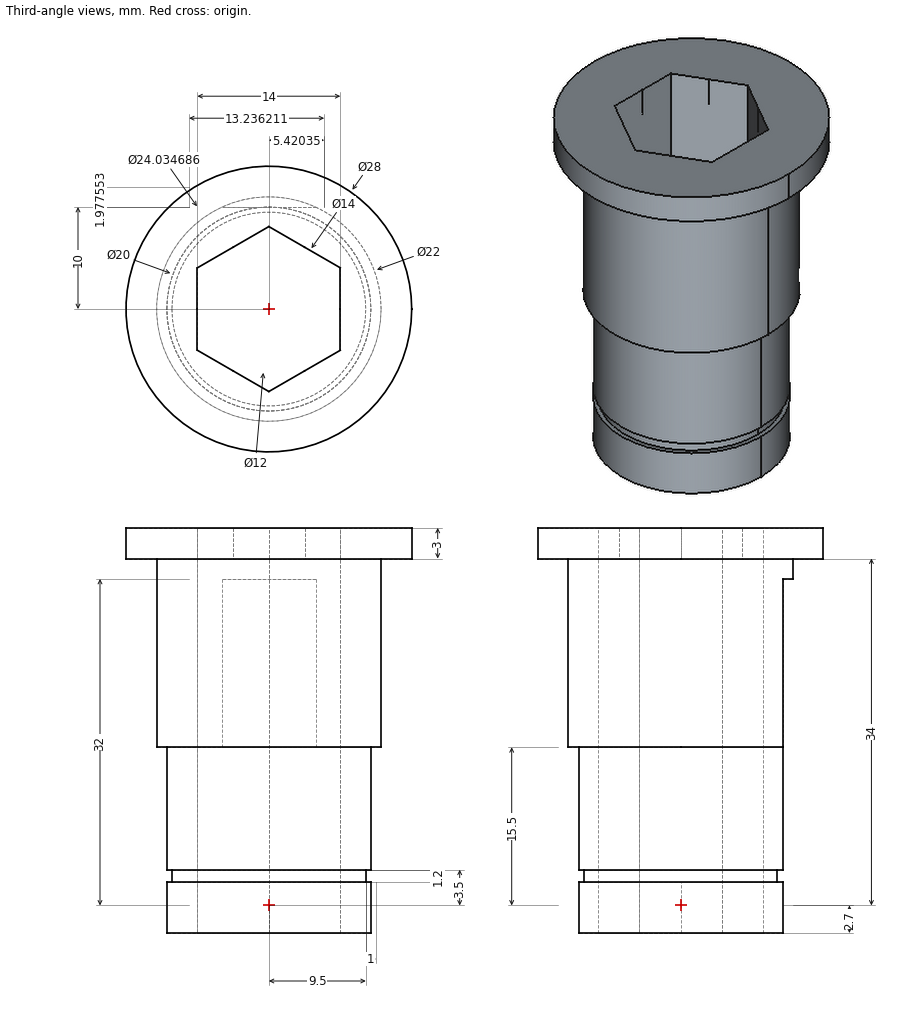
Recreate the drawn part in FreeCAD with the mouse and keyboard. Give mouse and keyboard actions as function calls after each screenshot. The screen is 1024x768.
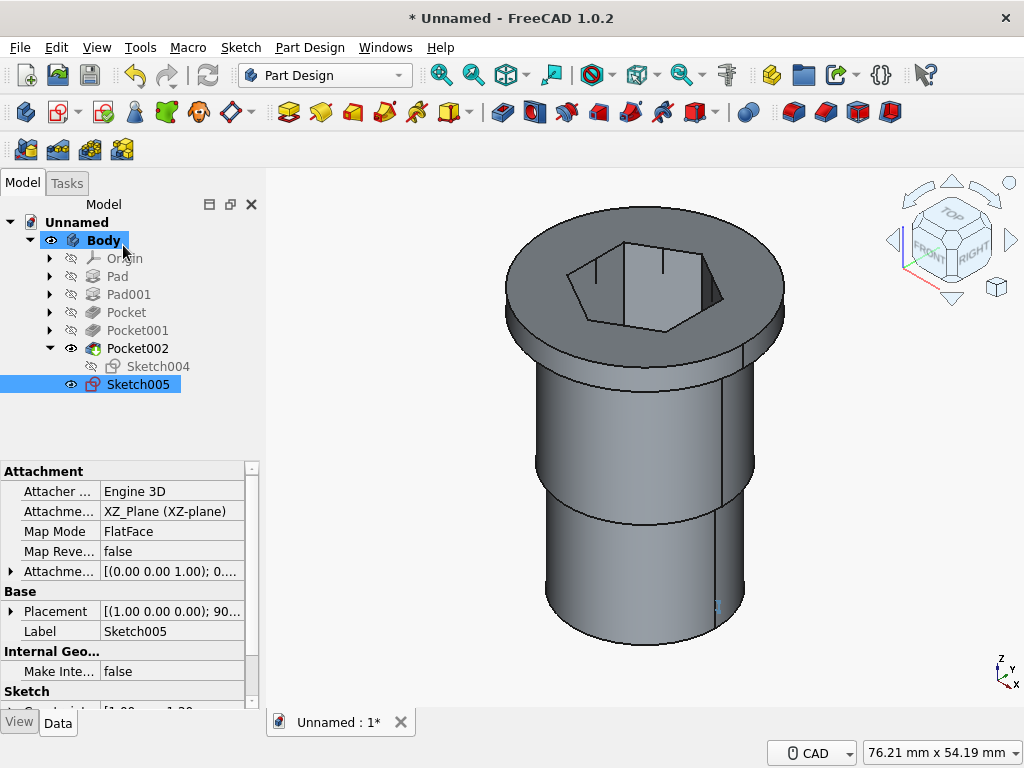
click(568, 112)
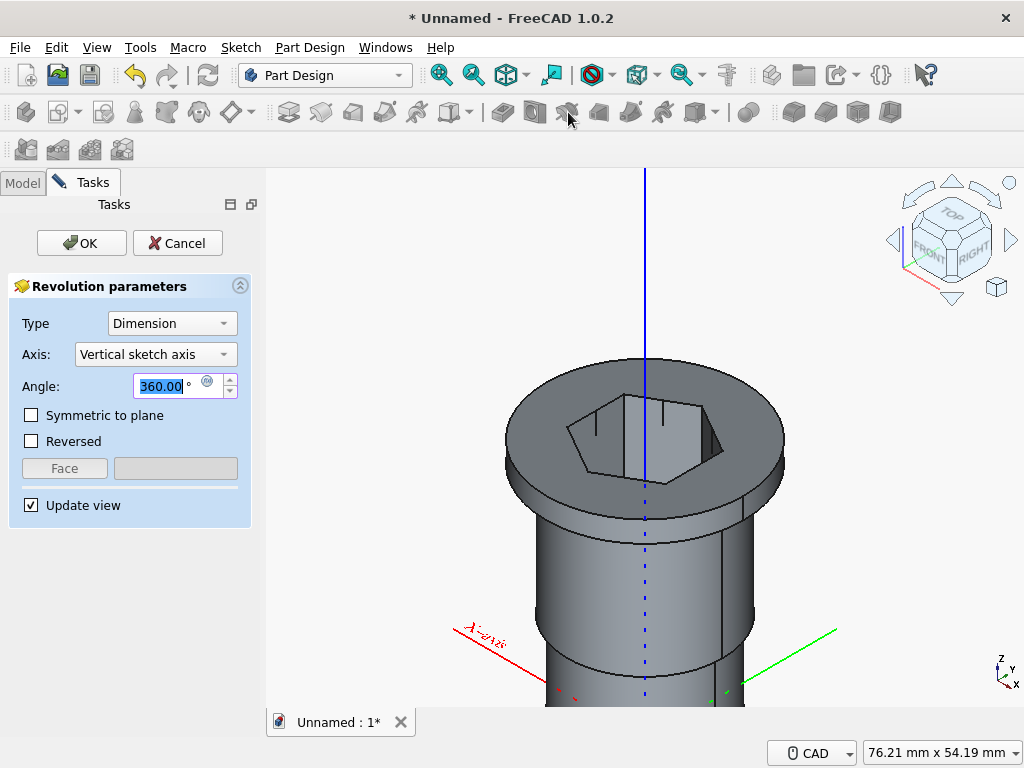
click(82, 243)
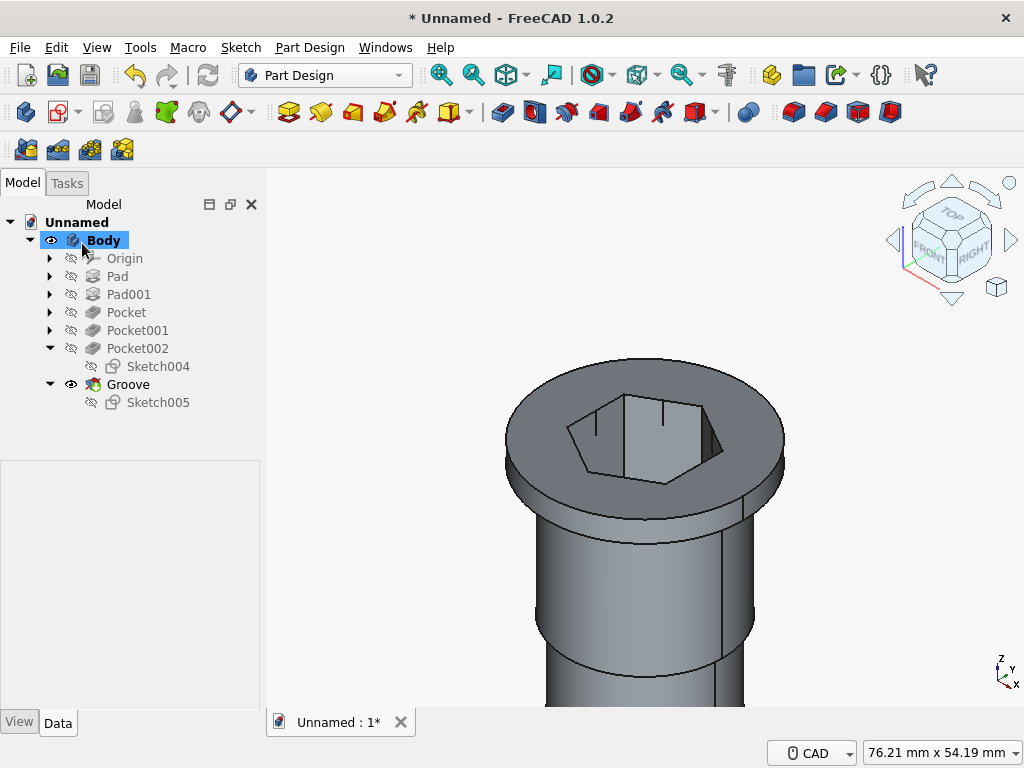
click(442, 76)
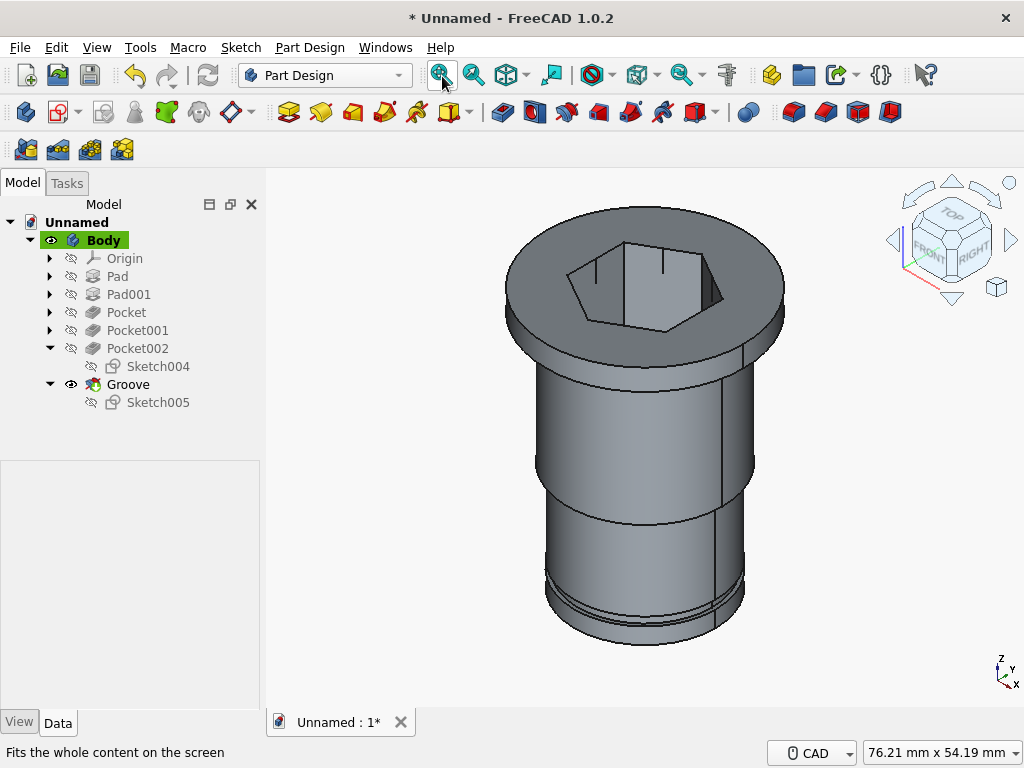
click(50, 258)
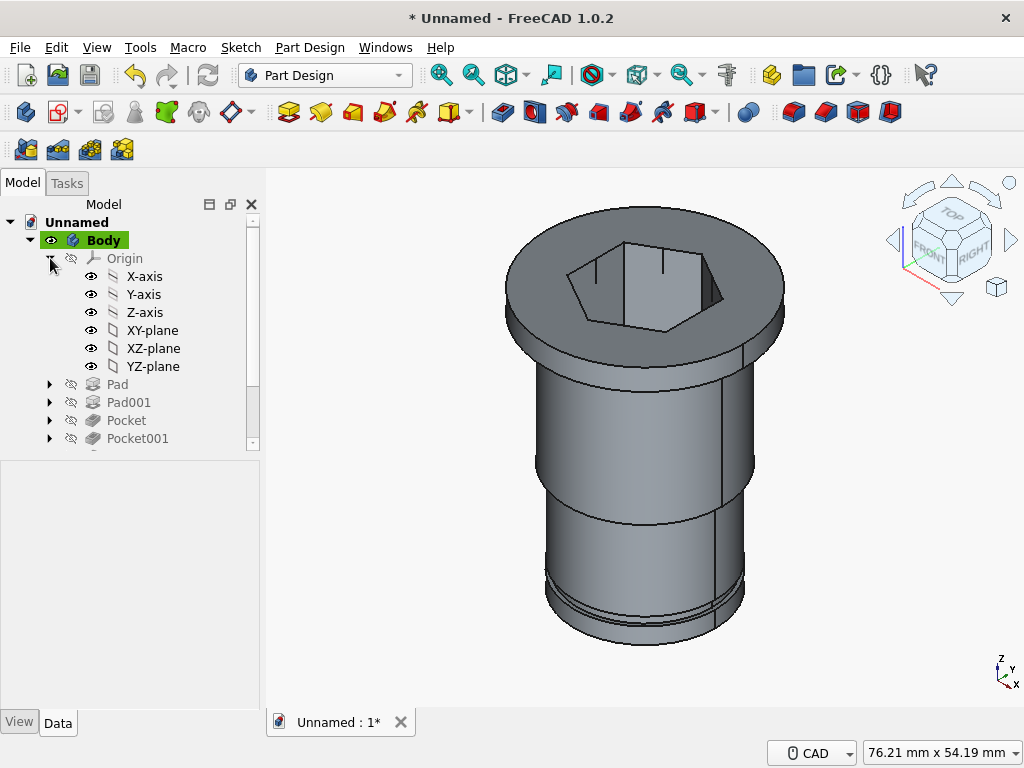
click(136, 330)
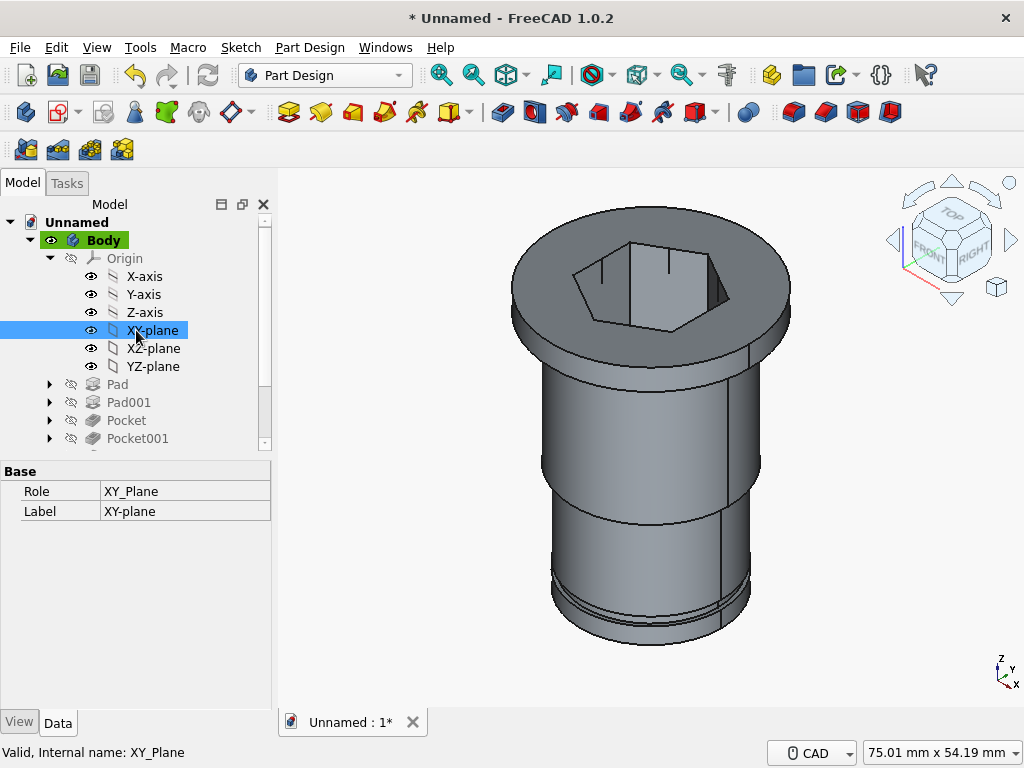
click(232, 112)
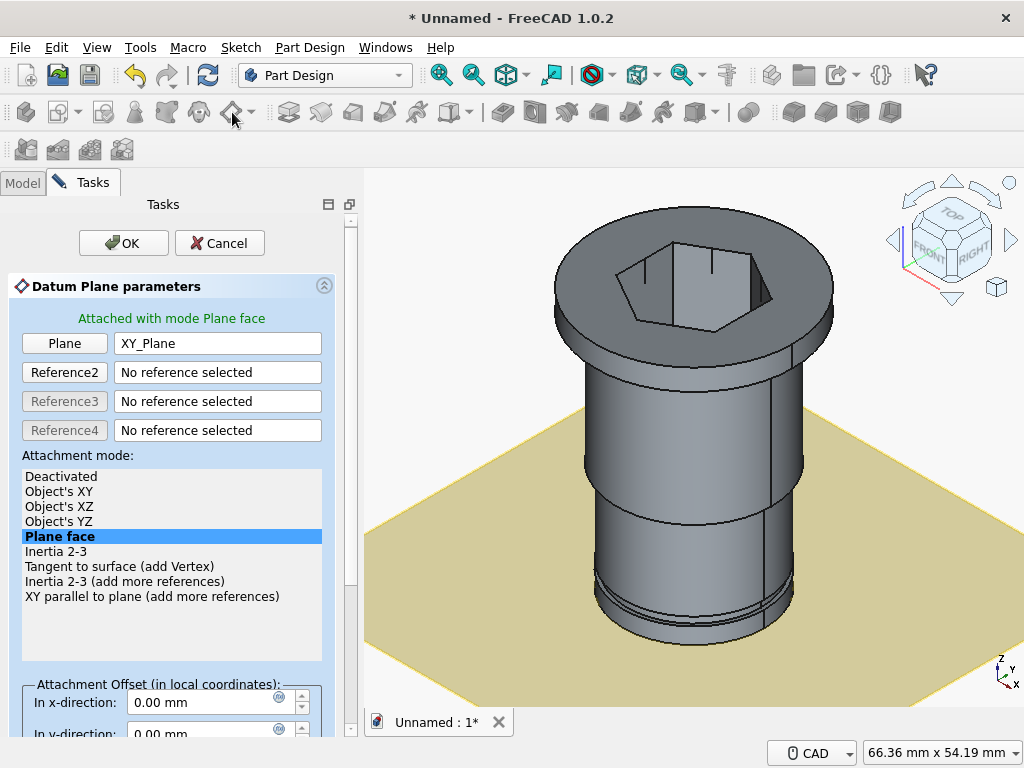
scroll(351, 475, down, 2)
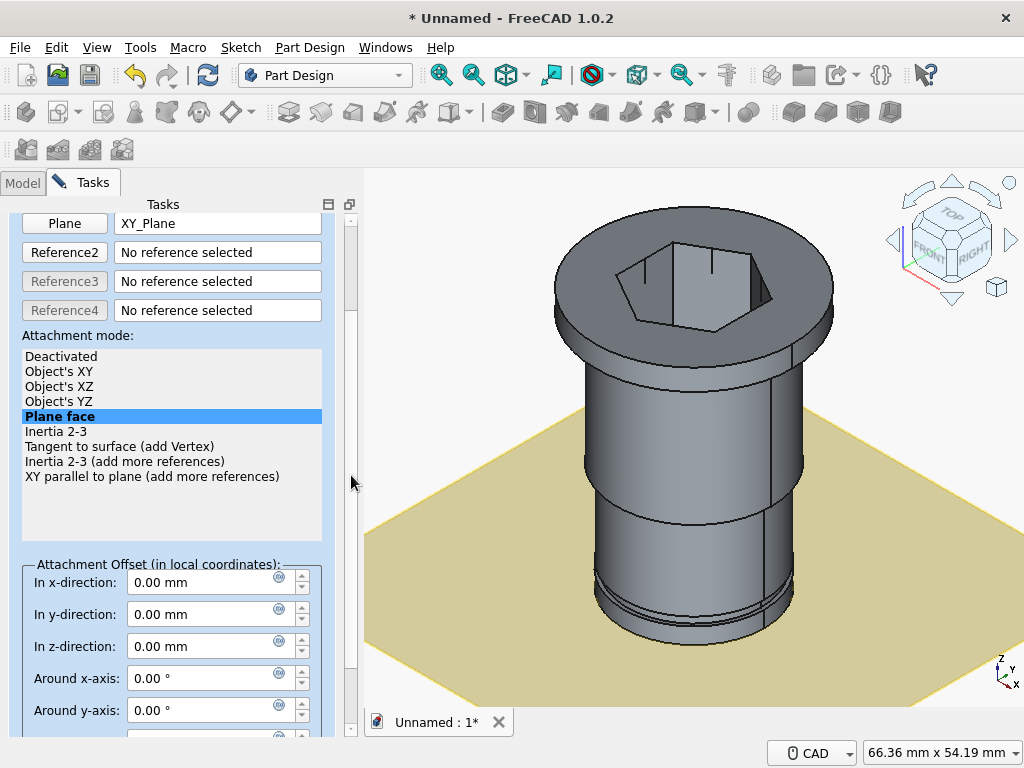
triple_click(210, 646)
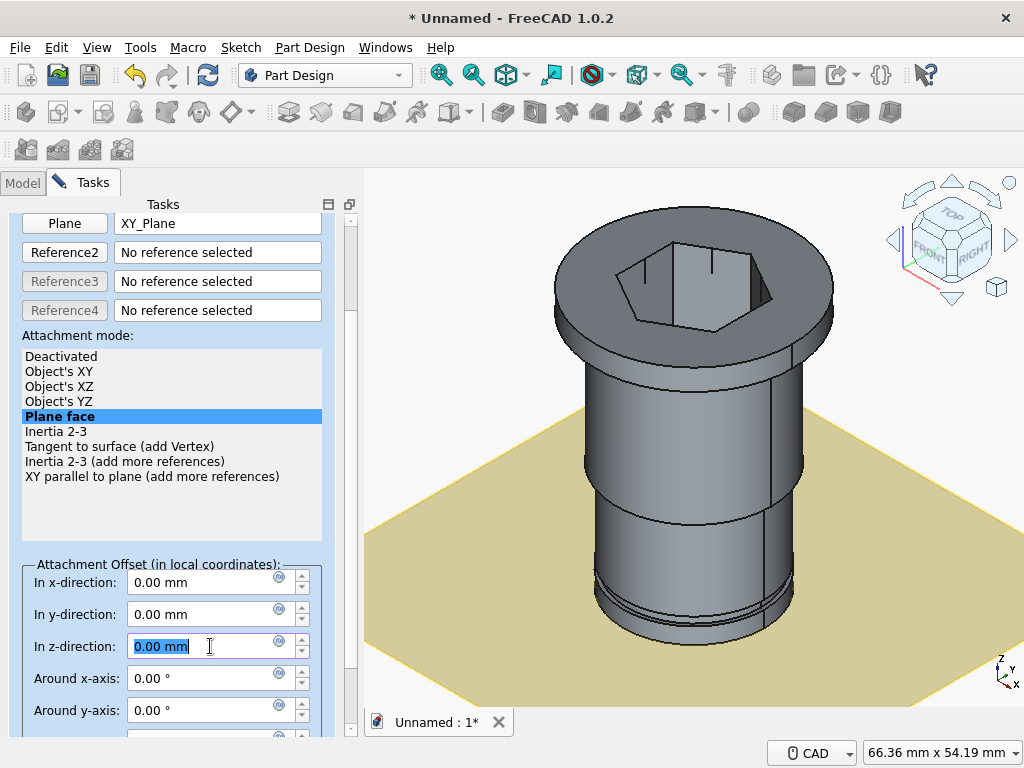
text(-2.7)
key(Tab)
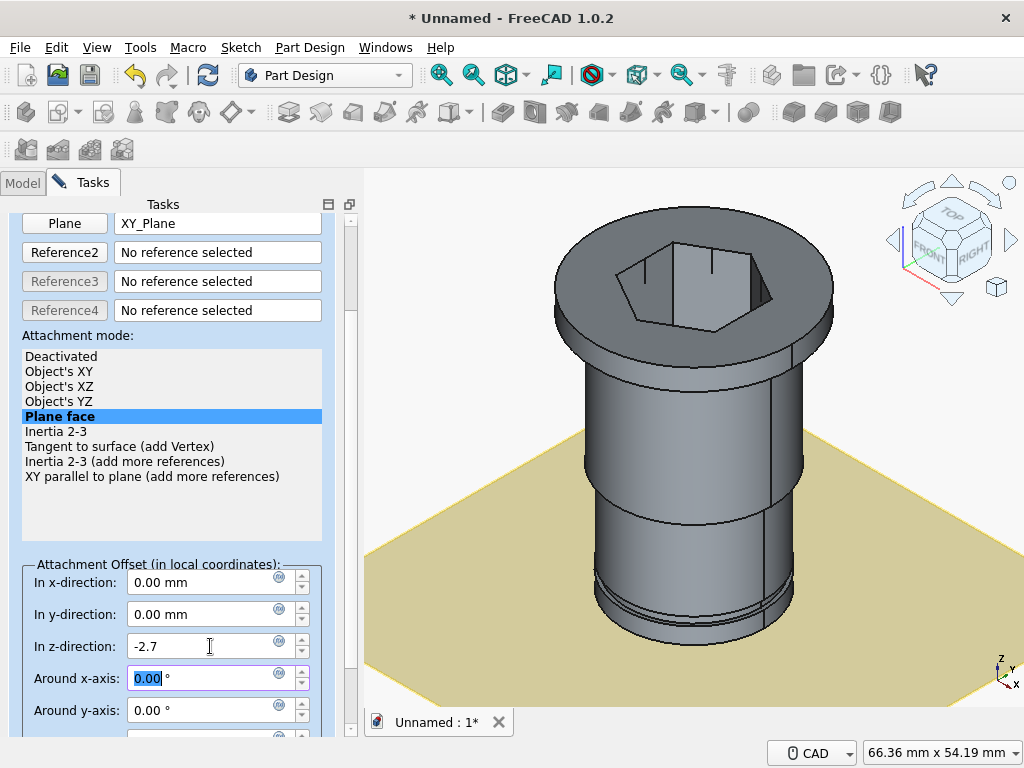
scroll(351, 475, up, 3)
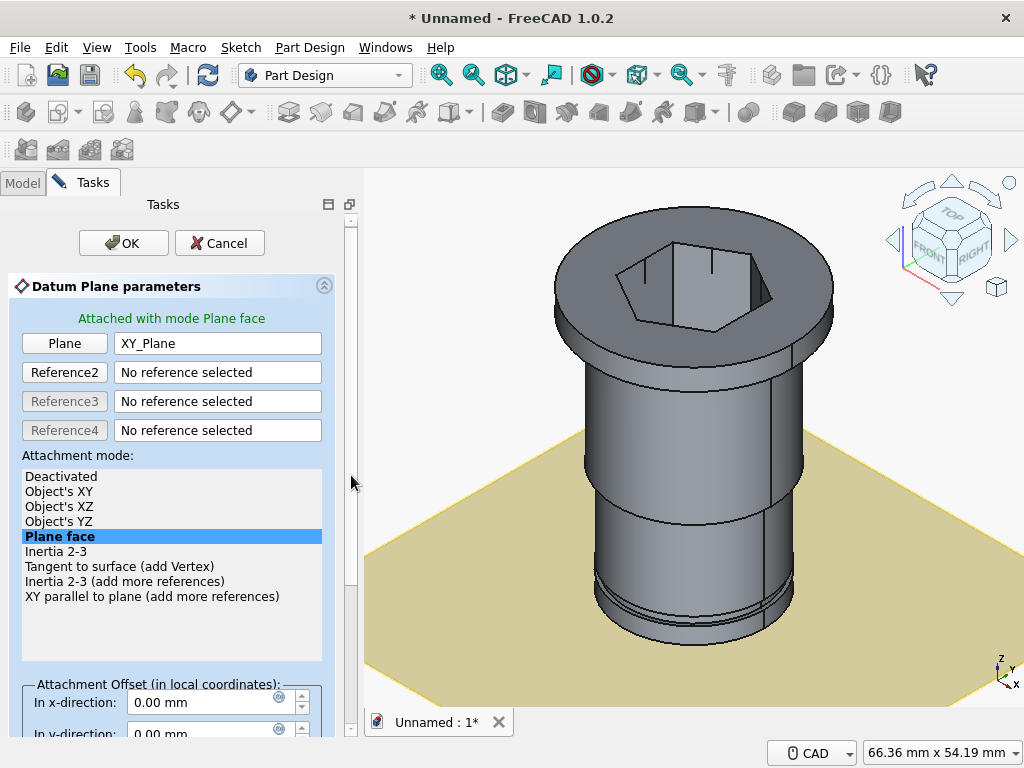
click(124, 243)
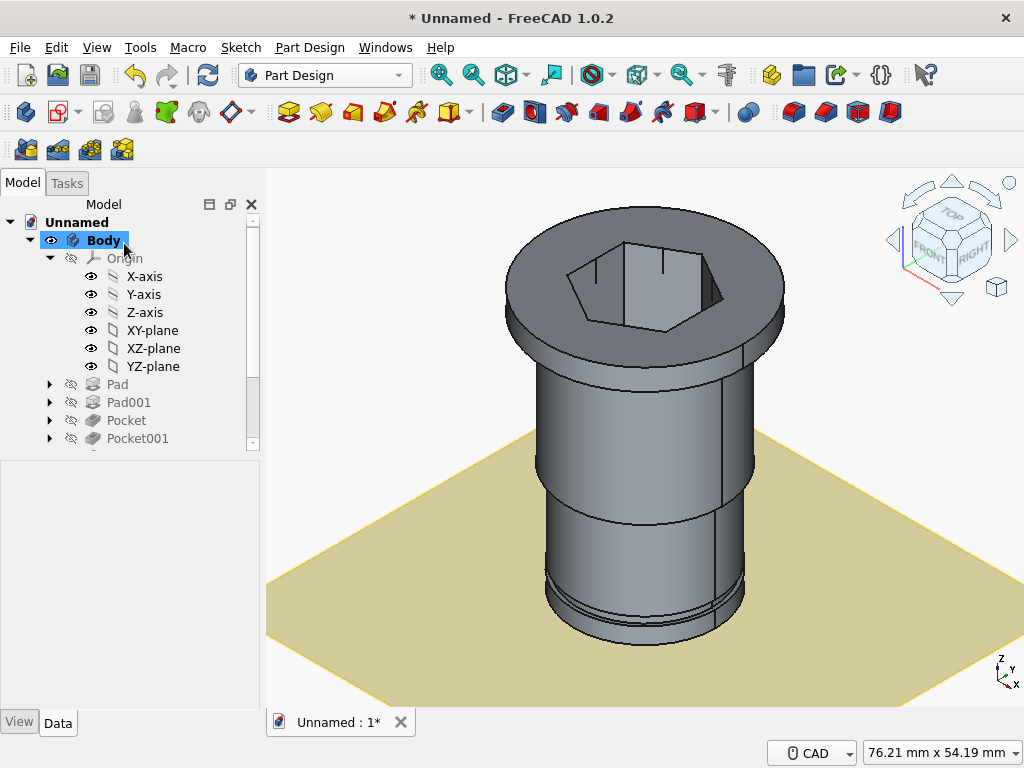
scroll(100, 326, down, 3)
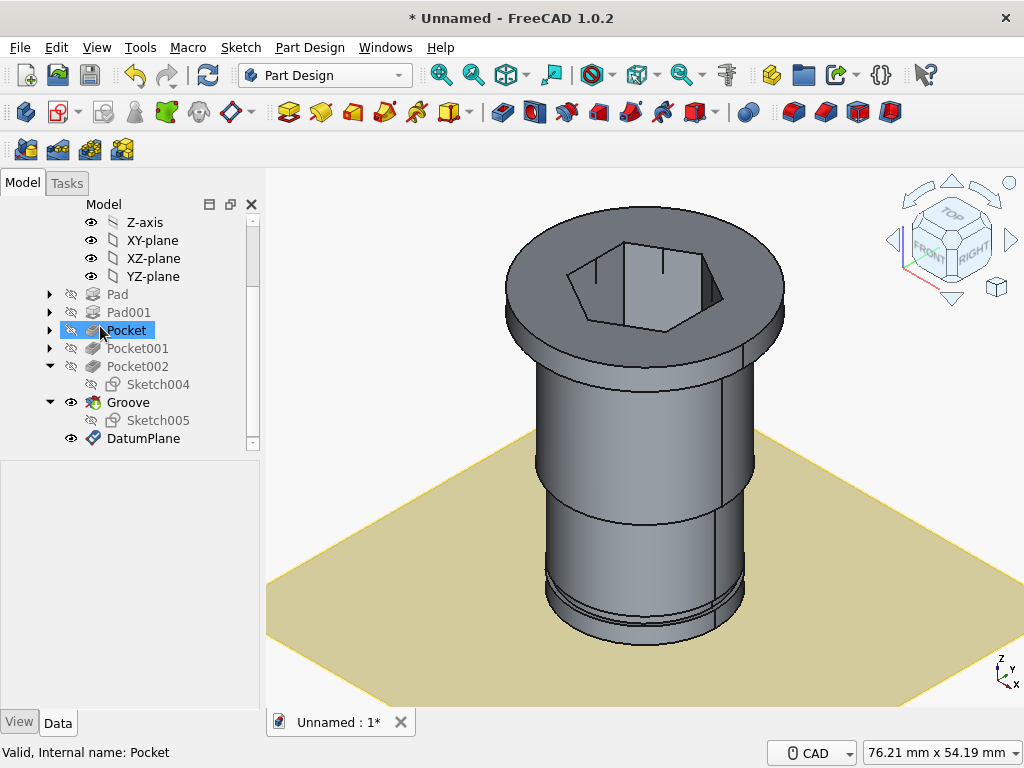
click(116, 438)